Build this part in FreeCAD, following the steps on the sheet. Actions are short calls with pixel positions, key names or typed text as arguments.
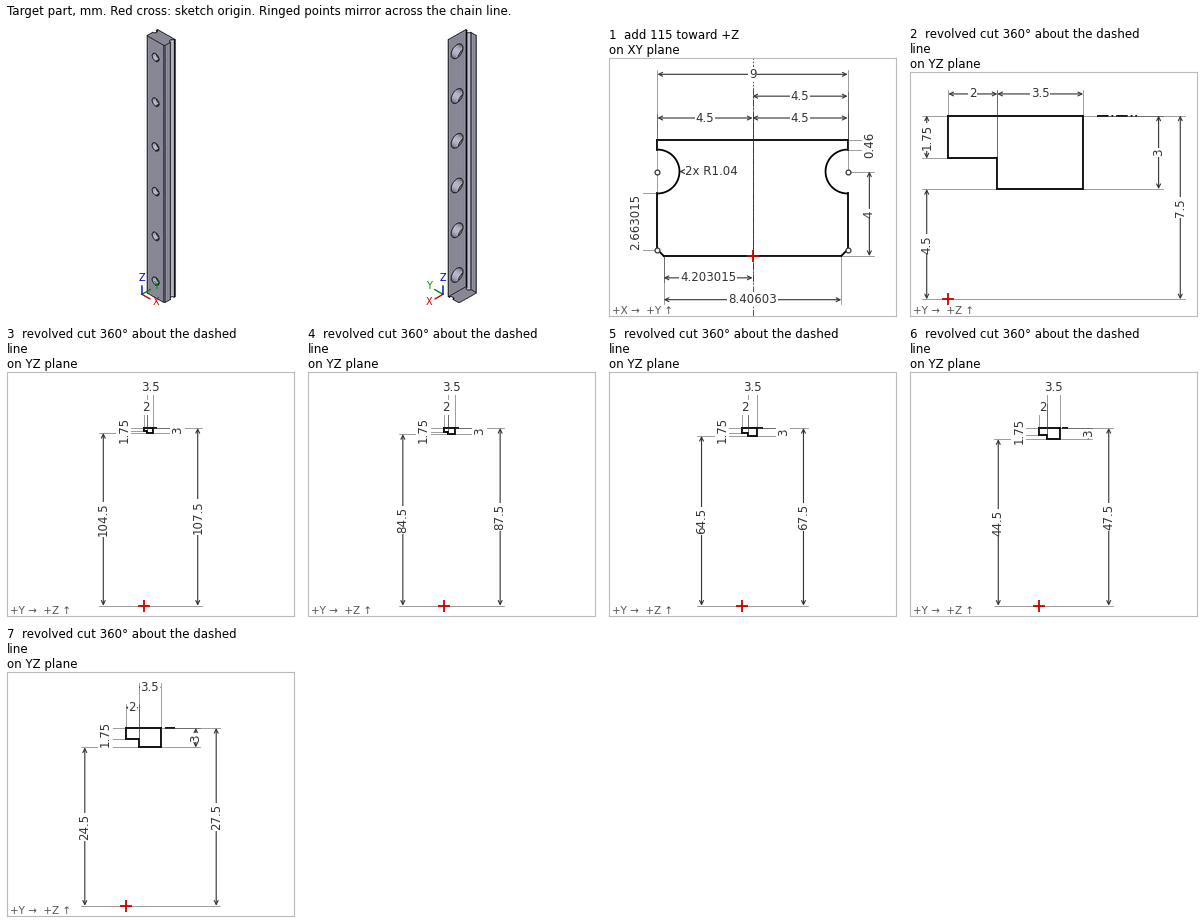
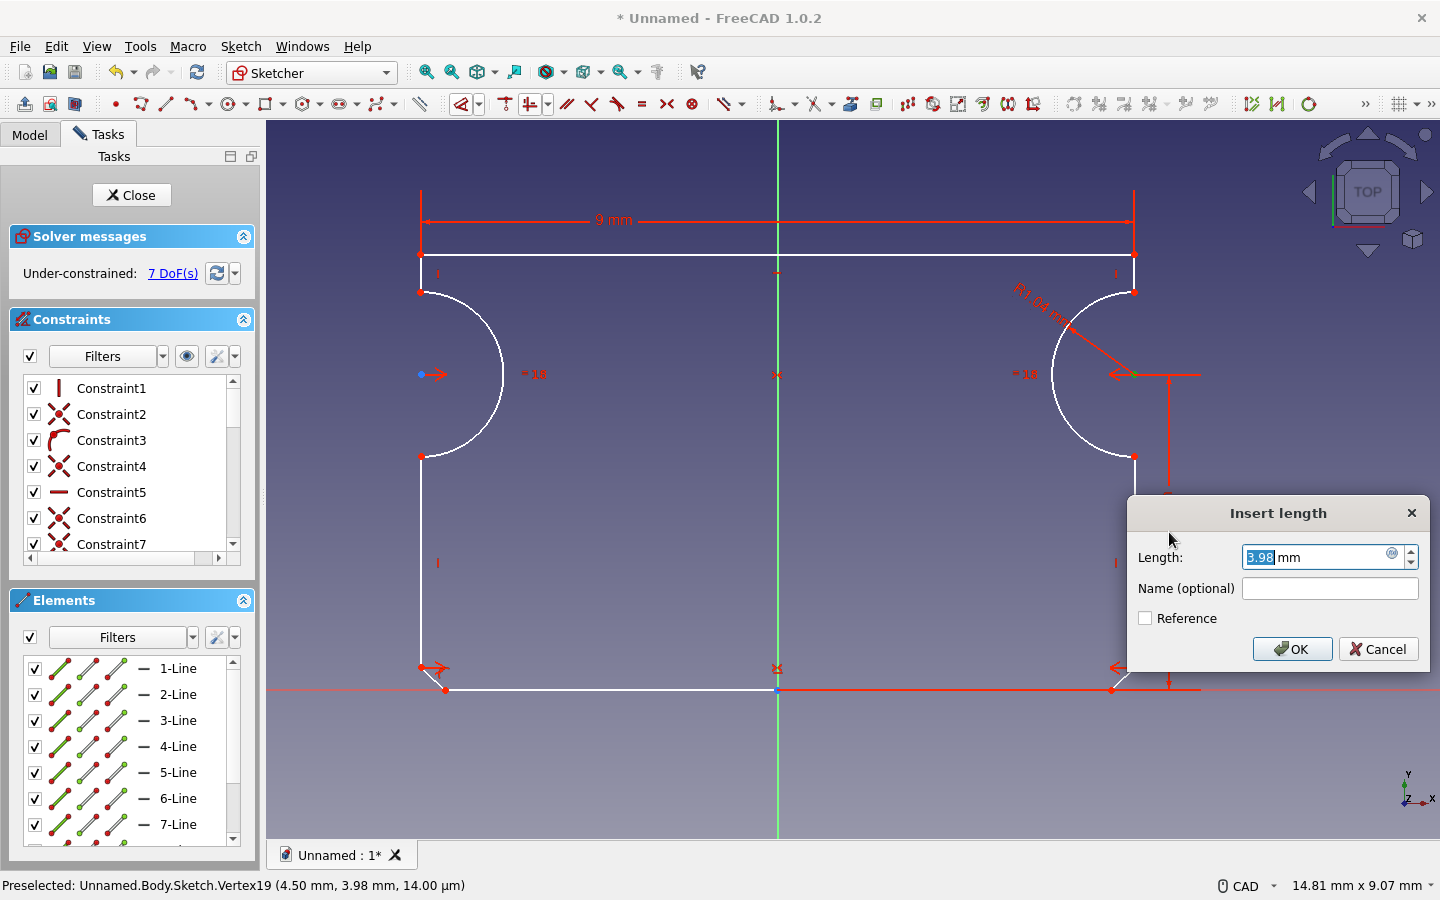
text(4)
key(Return)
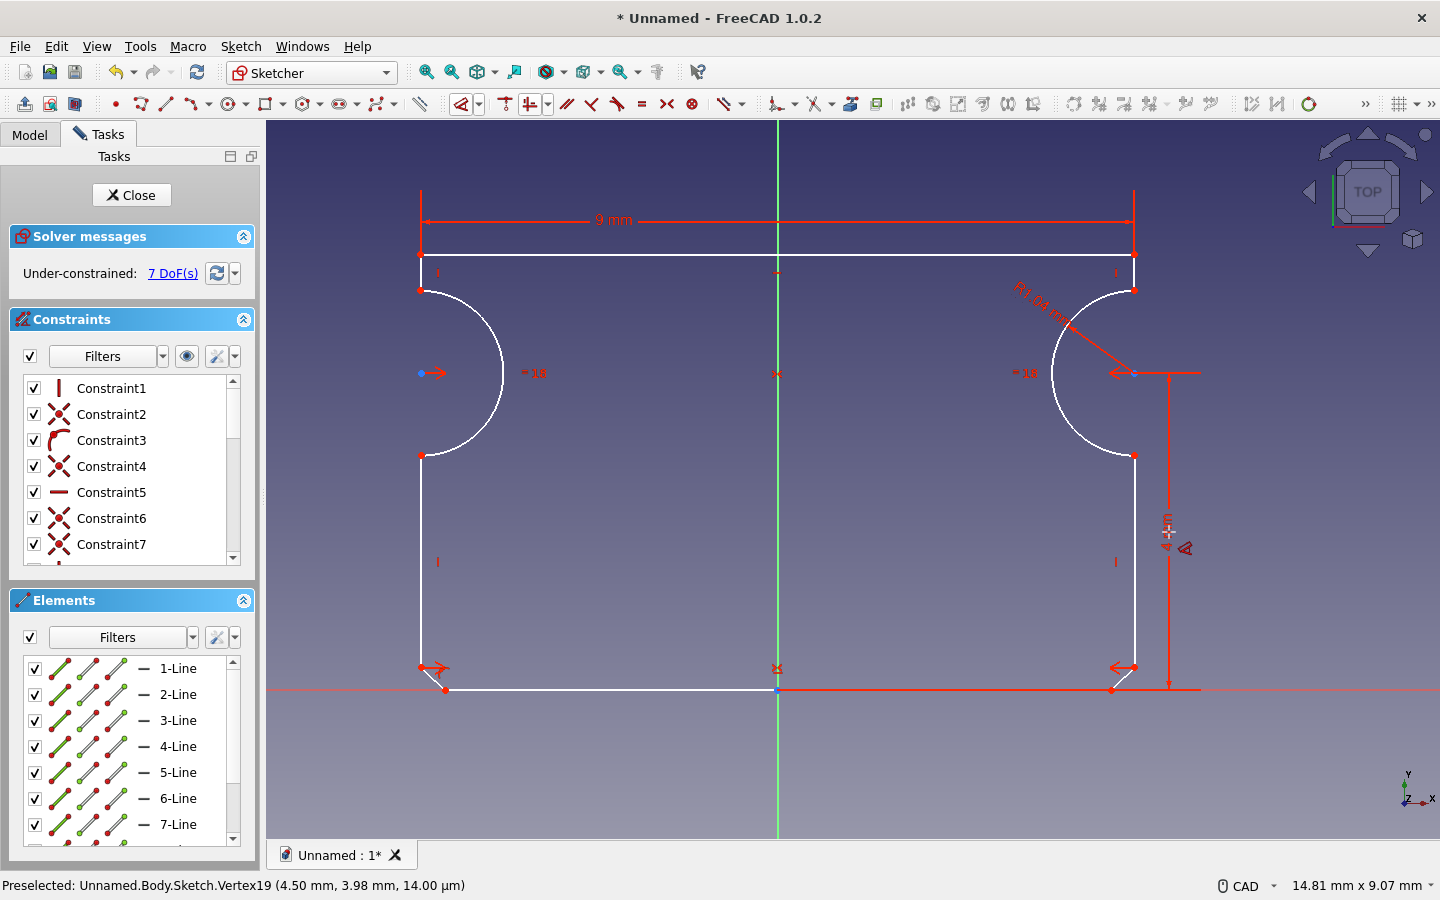
scroll(1134, 280, up, 2)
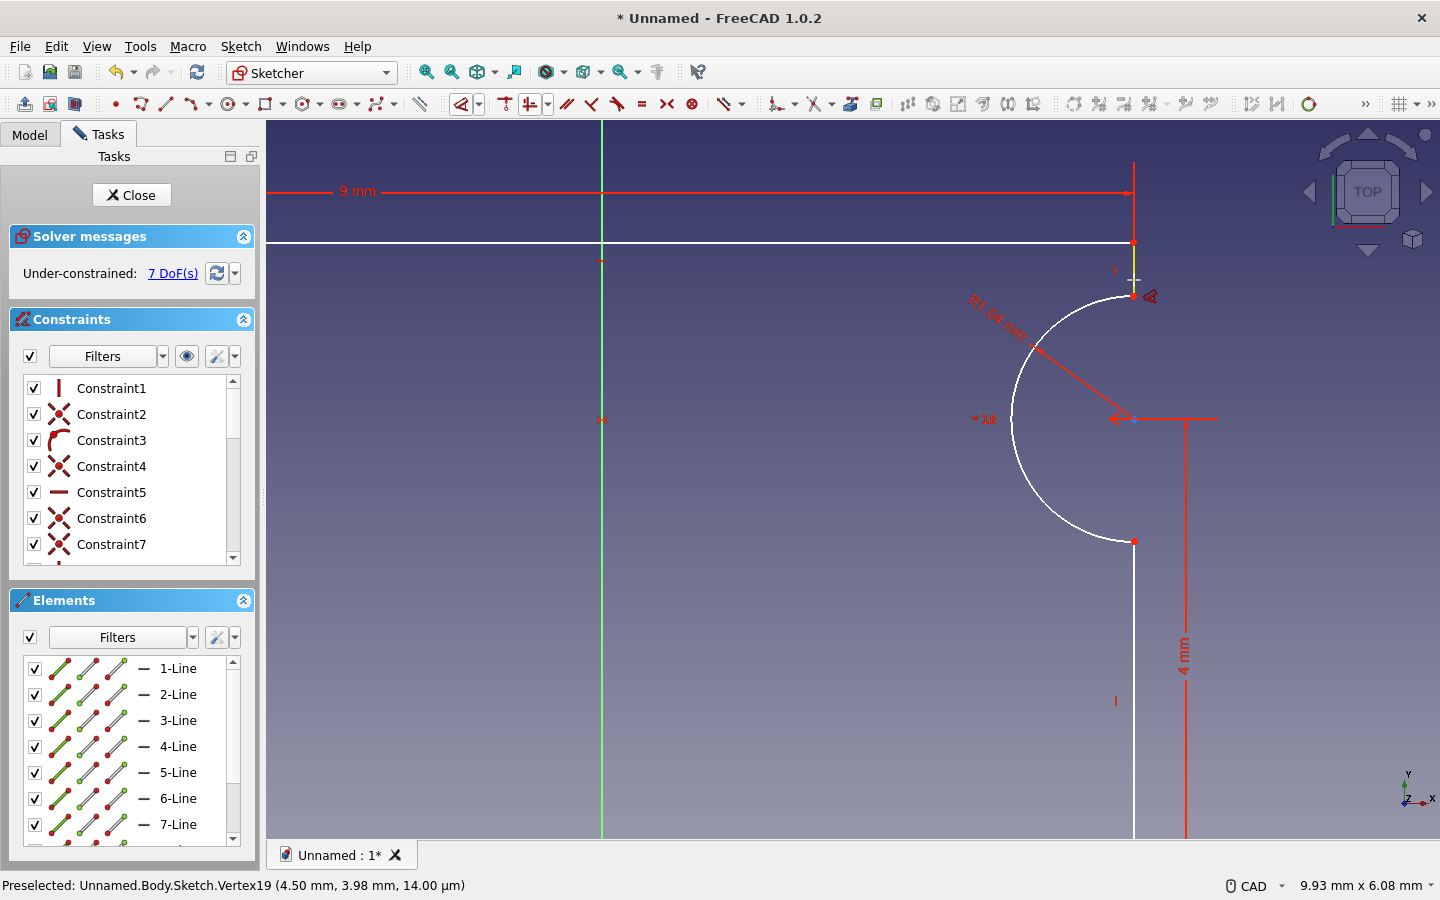
click(1134, 280)
click(1168, 269)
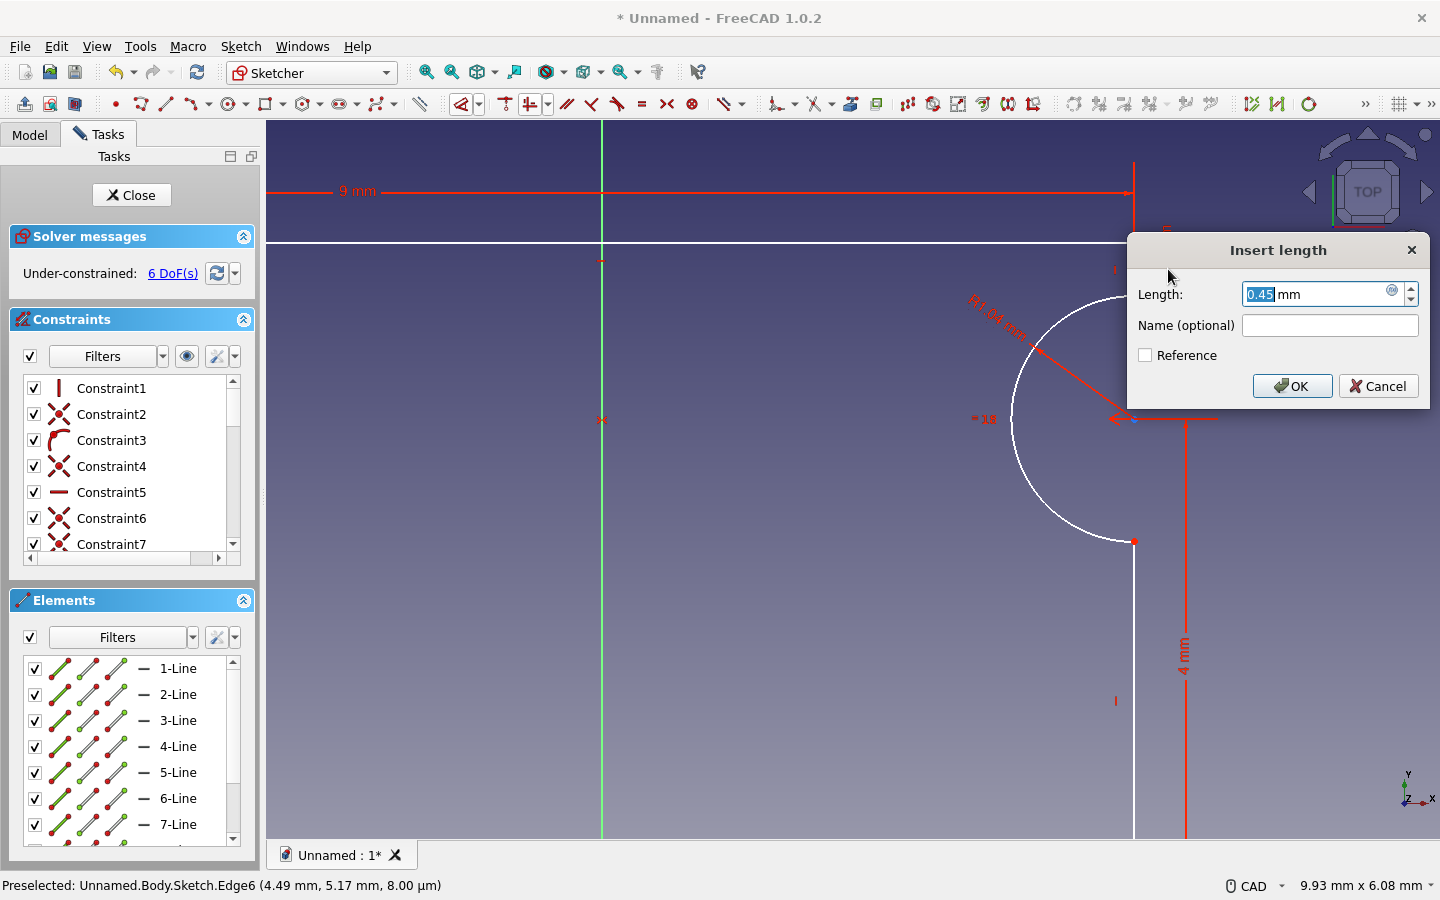
text(0.46)
key(Return)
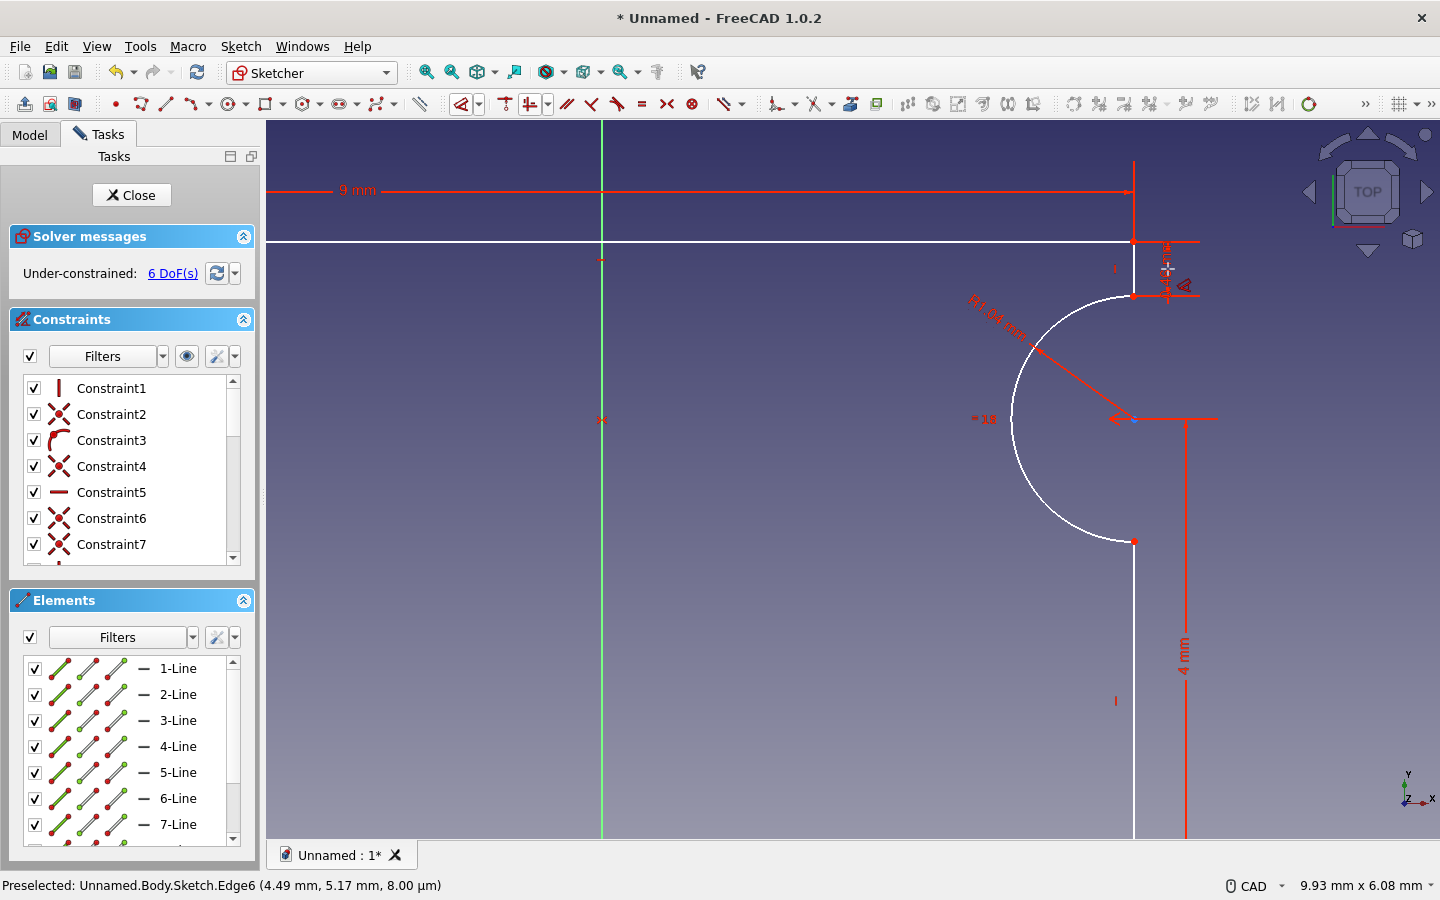
scroll(1155, 302, down, 2)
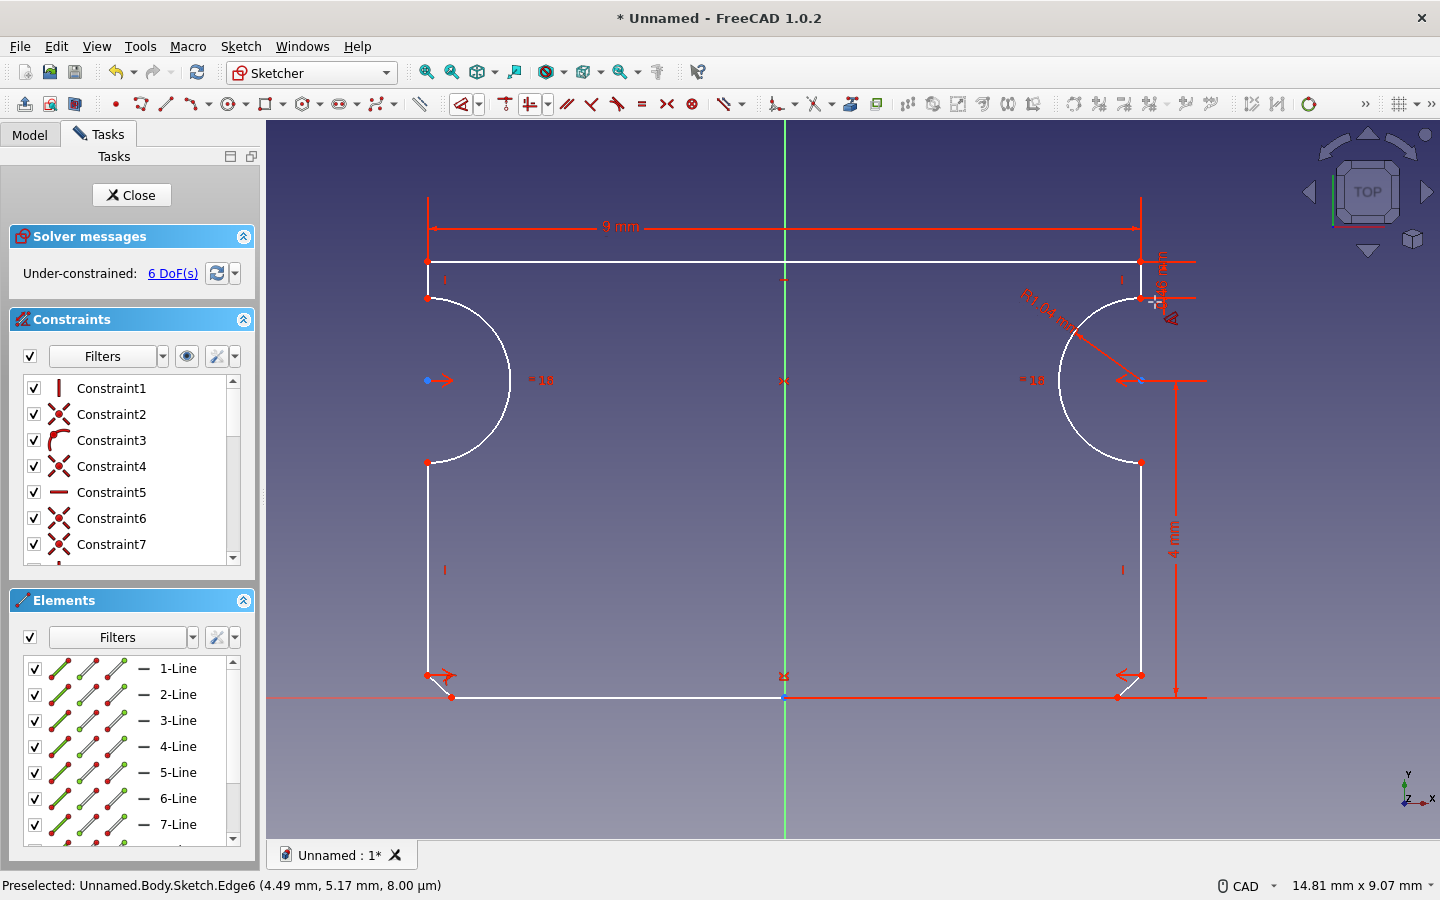
click(428, 463)
click(606, 732)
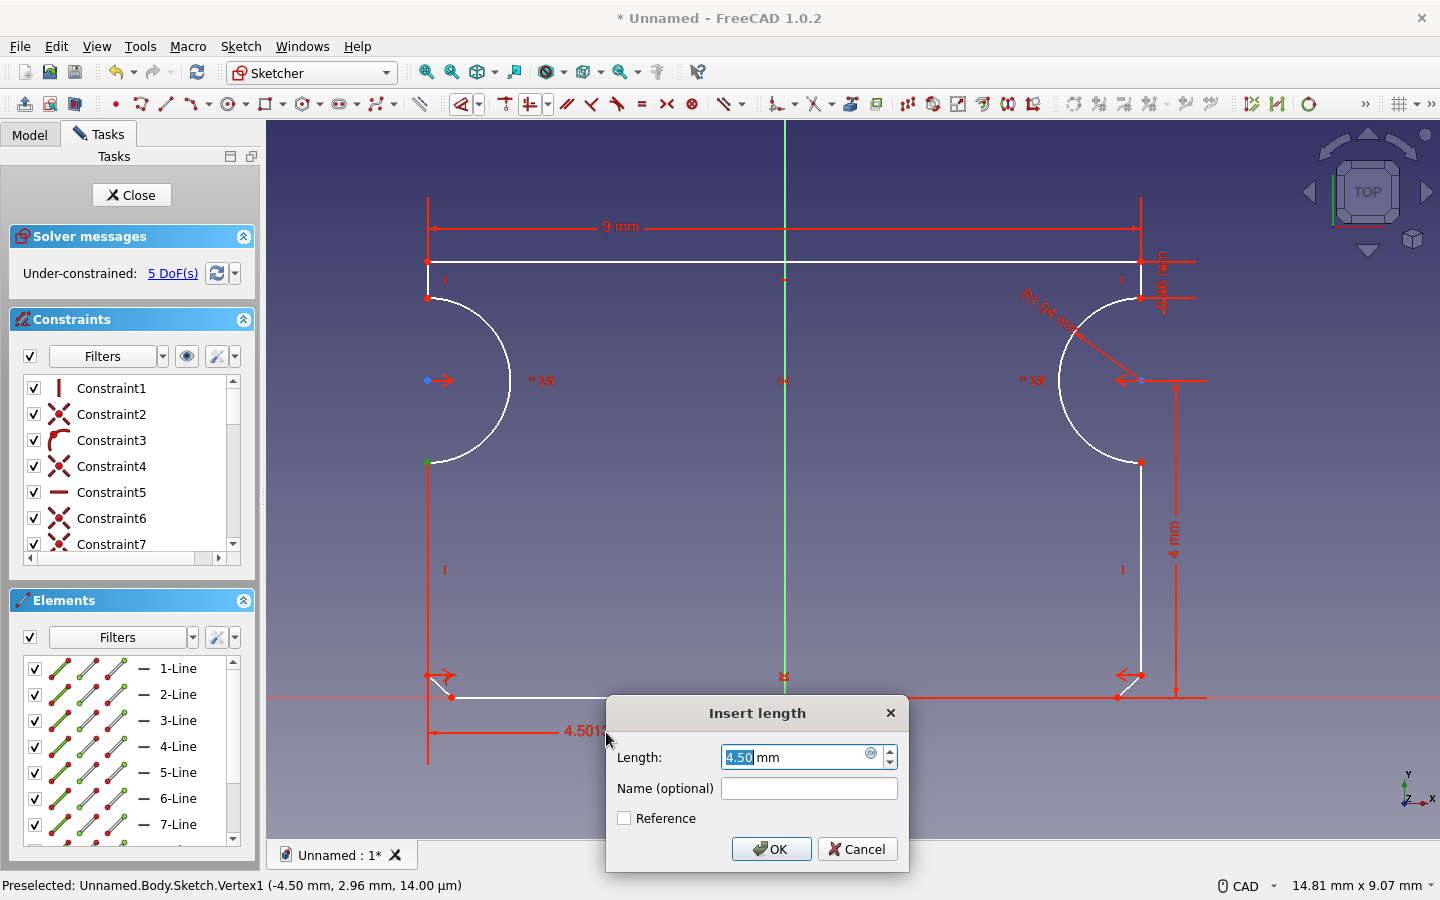
text(4.5)
key(Return)